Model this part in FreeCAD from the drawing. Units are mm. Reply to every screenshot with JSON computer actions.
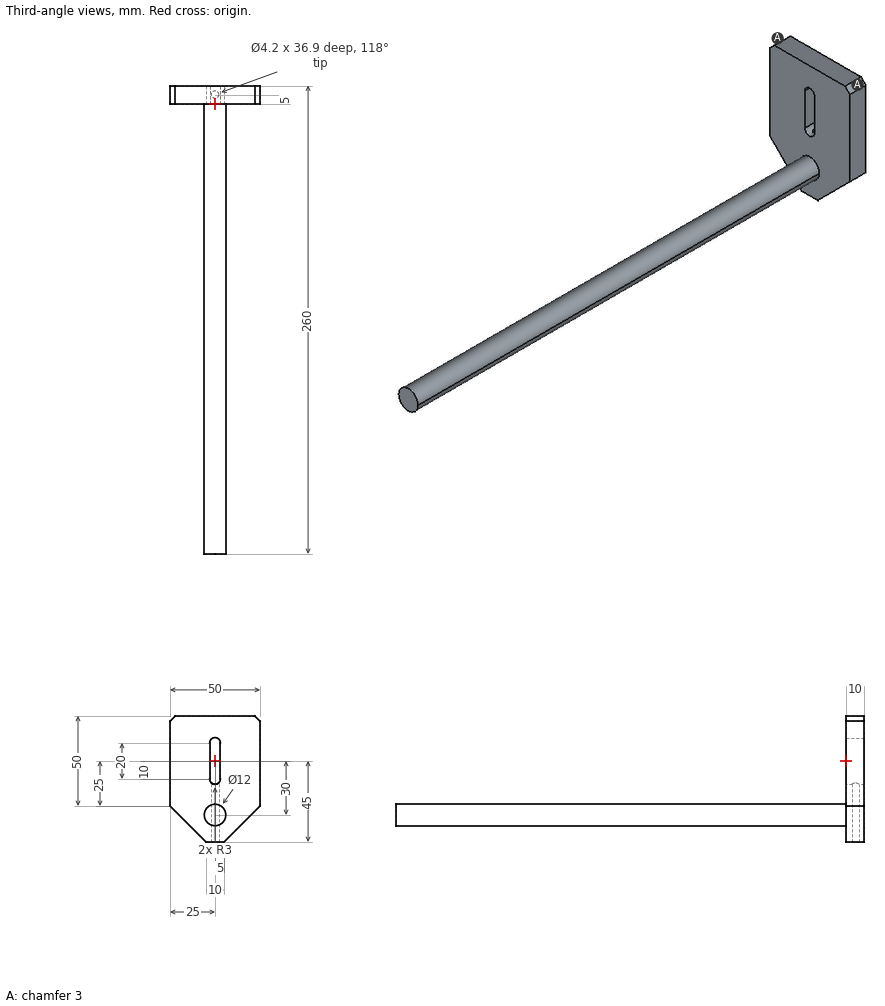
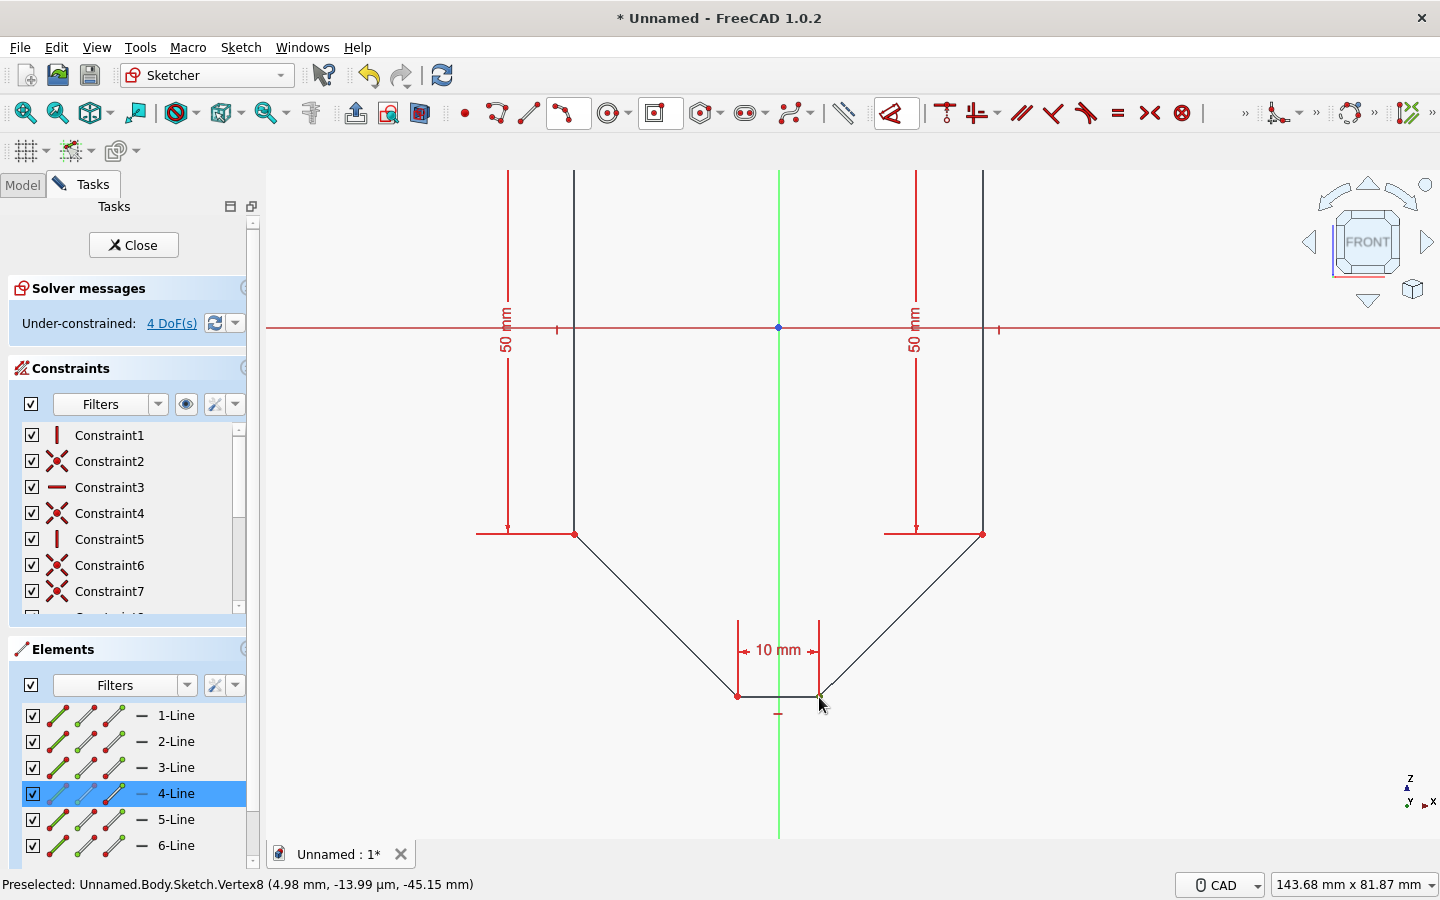
{"action": "left_click", "coordinate": [914, 114]}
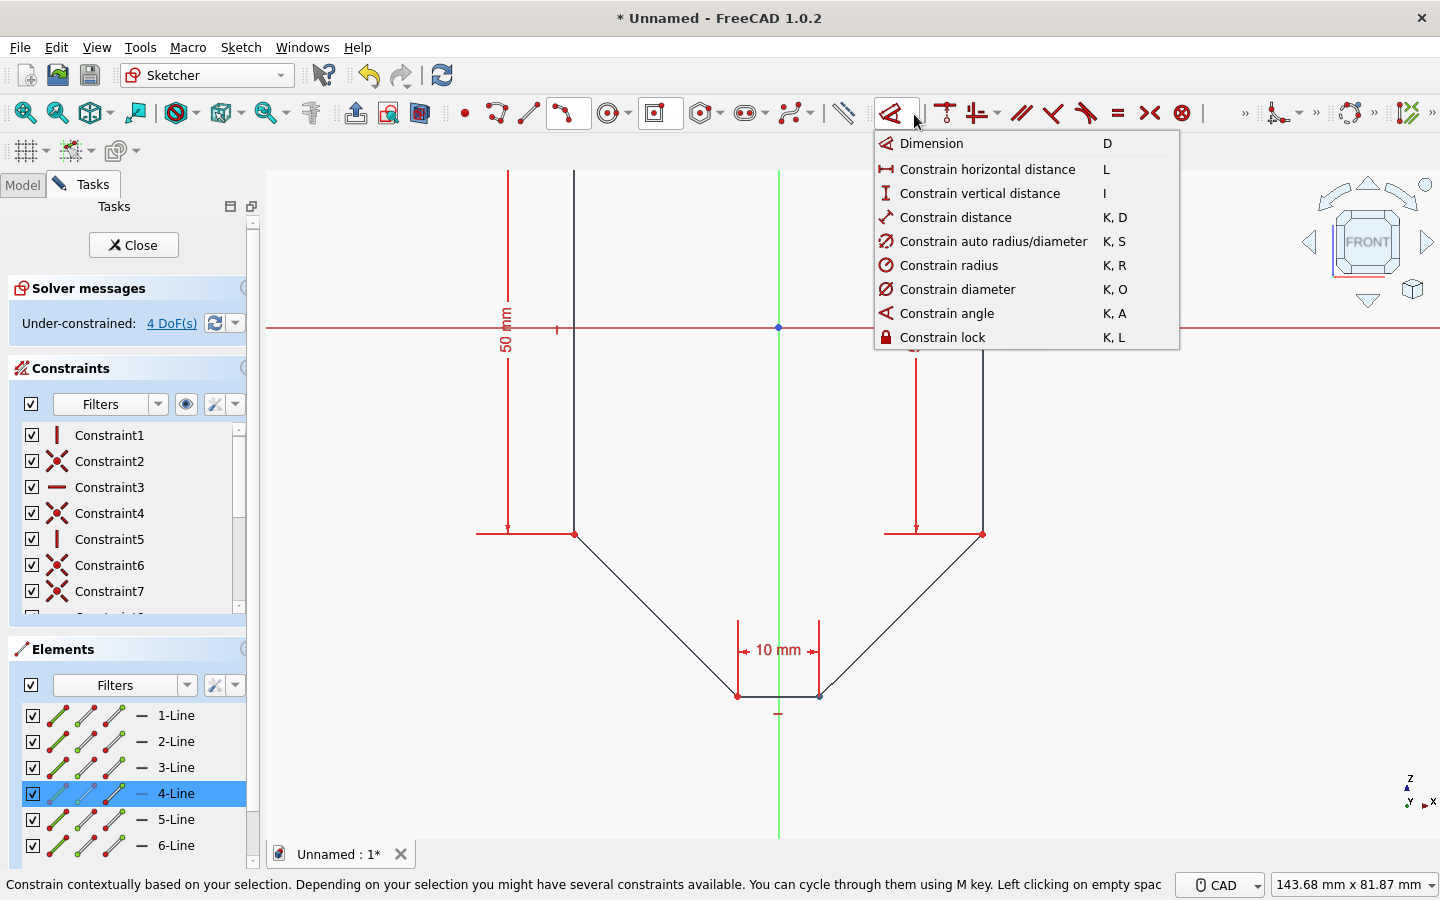
{"action": "left_click", "coordinate": [1027, 169]}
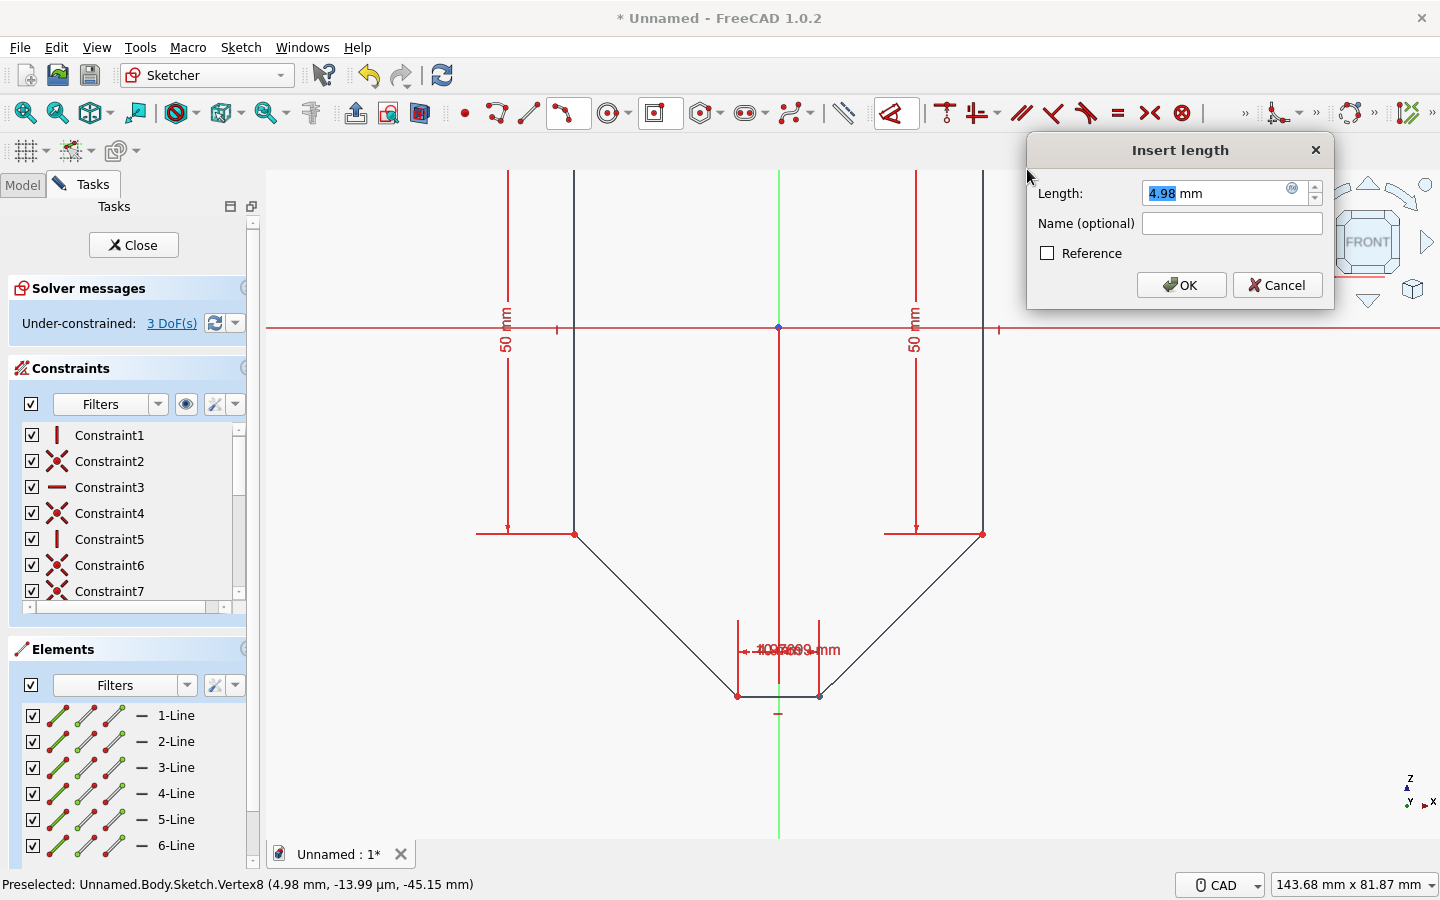
{"action": "type", "text": "5"}
{"action": "key", "text": "Return"}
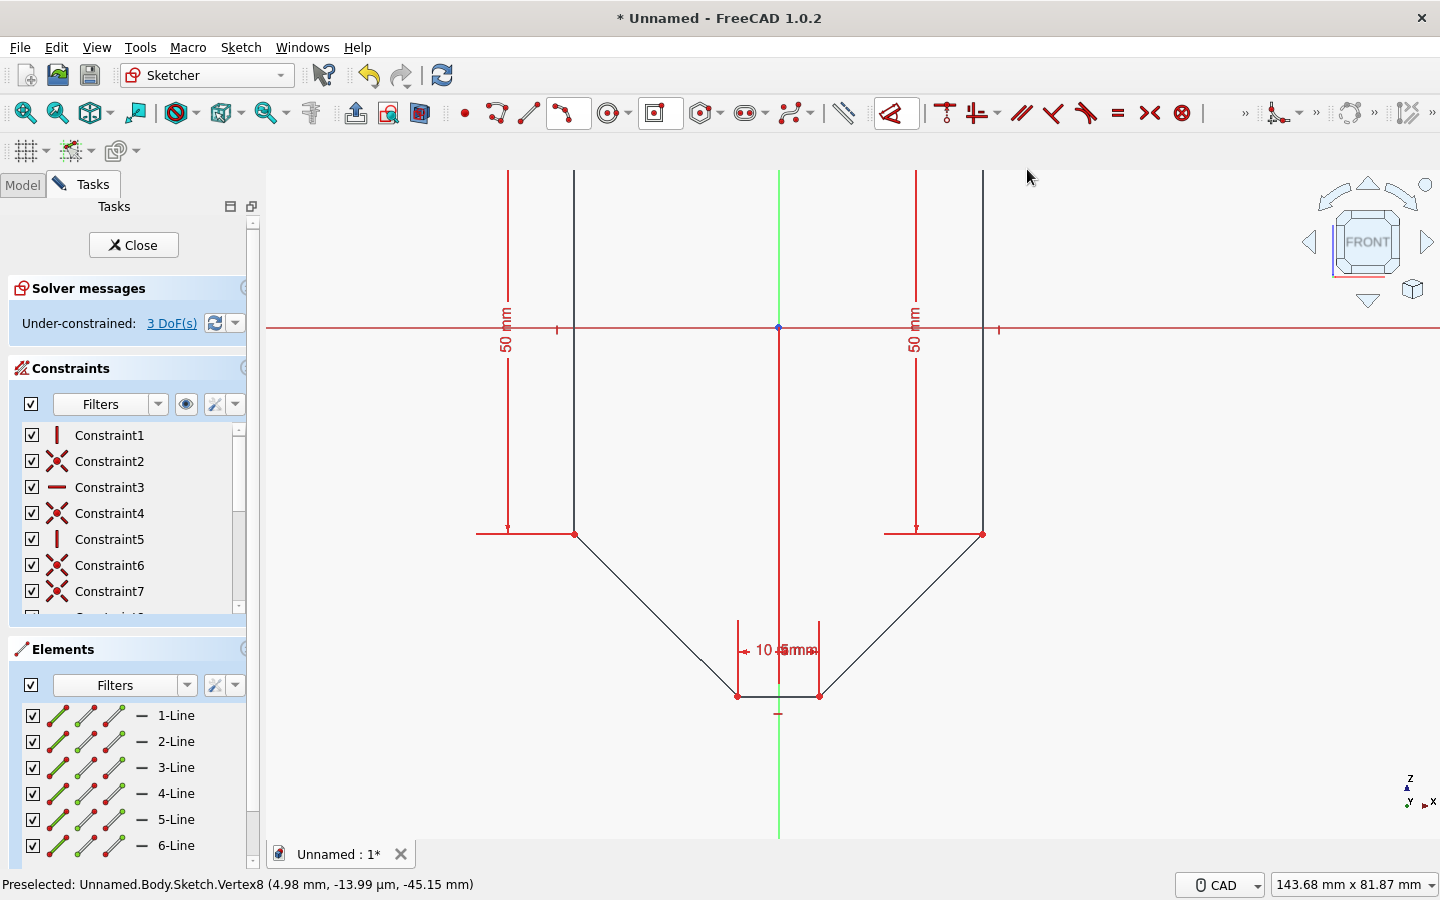
{"action": "left_click", "coordinate": [574, 534]}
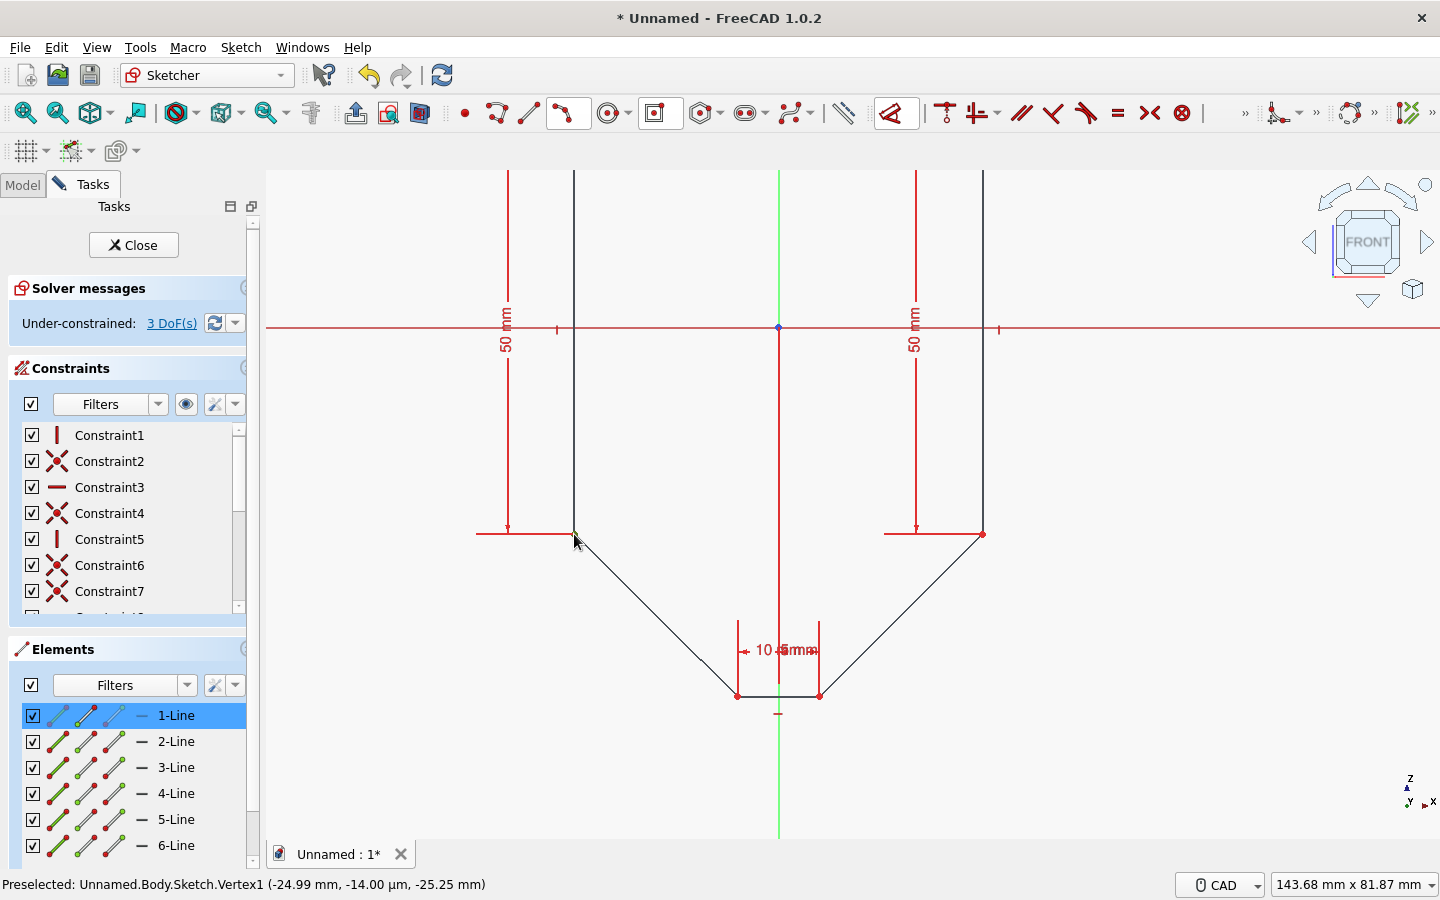
{"action": "key", "text": "l"}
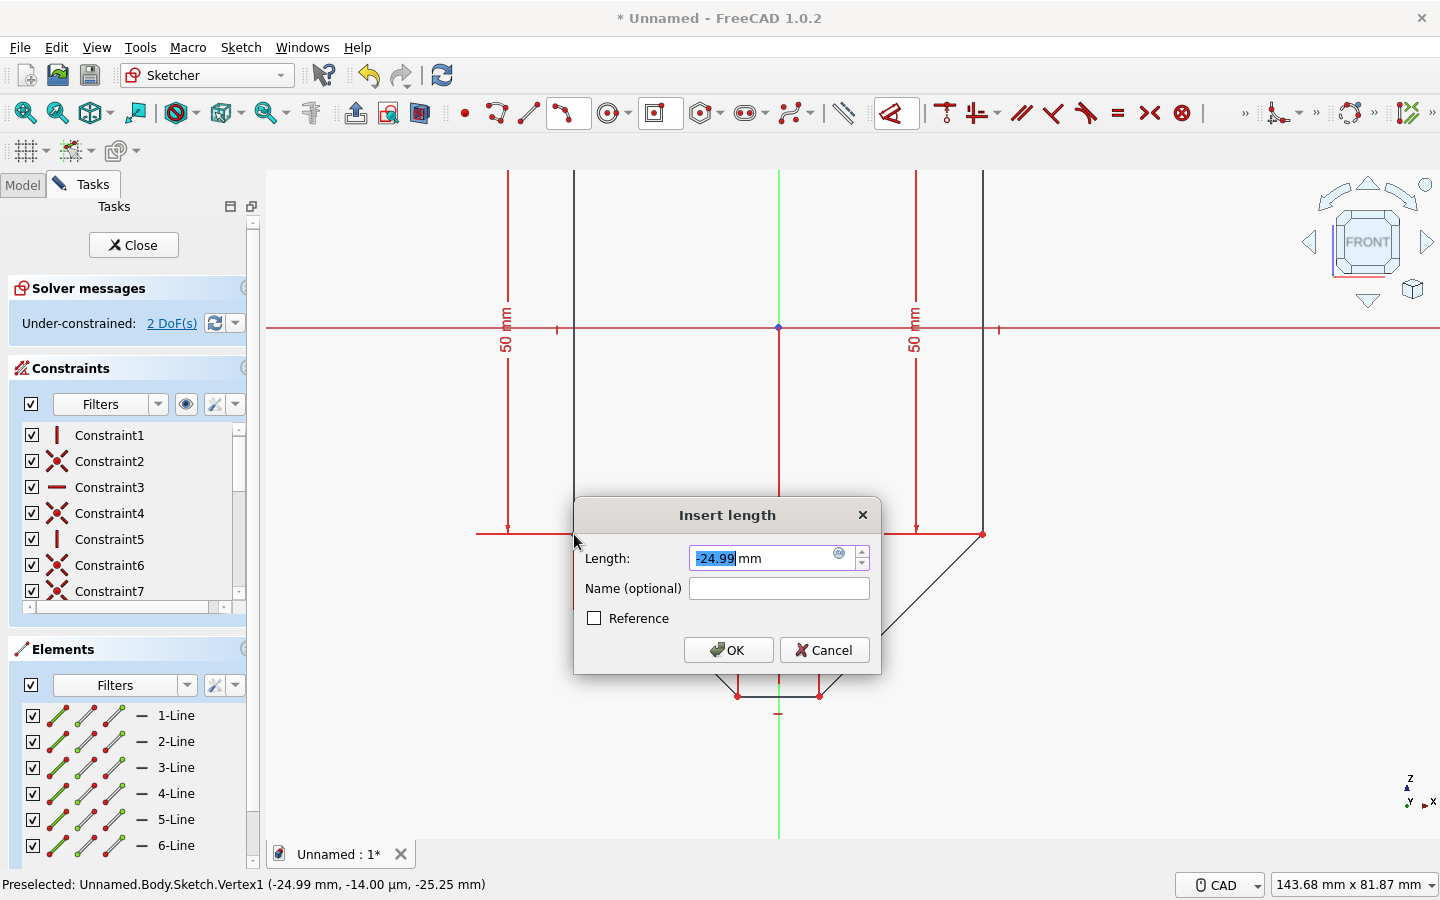
{"action": "type", "text": "-25"}
{"action": "key", "text": "Return"}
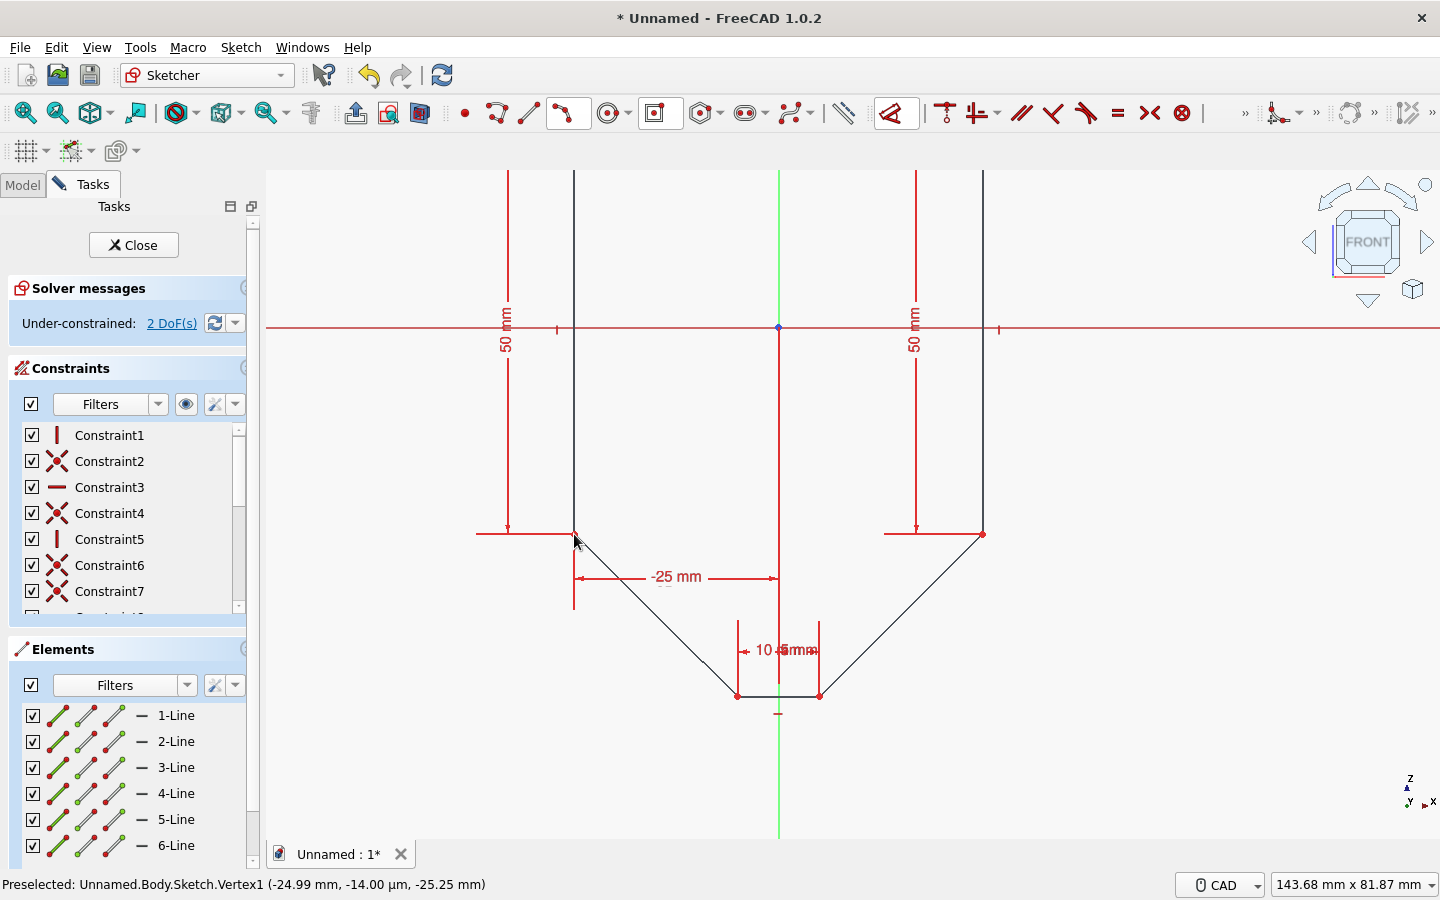
{"action": "left_click", "coordinate": [574, 534]}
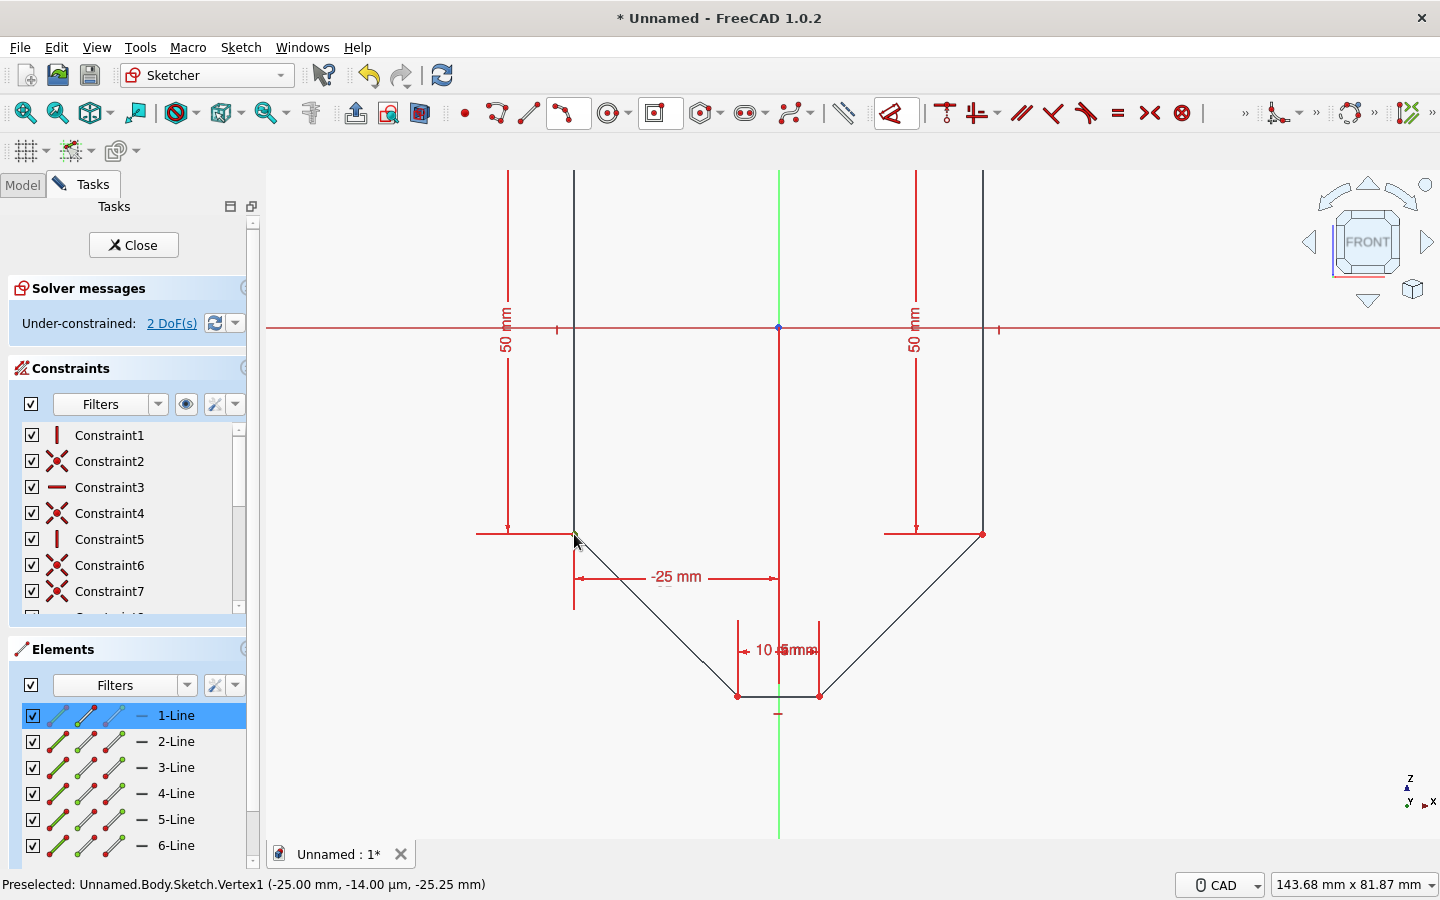
{"action": "left_click", "coordinate": [914, 114]}